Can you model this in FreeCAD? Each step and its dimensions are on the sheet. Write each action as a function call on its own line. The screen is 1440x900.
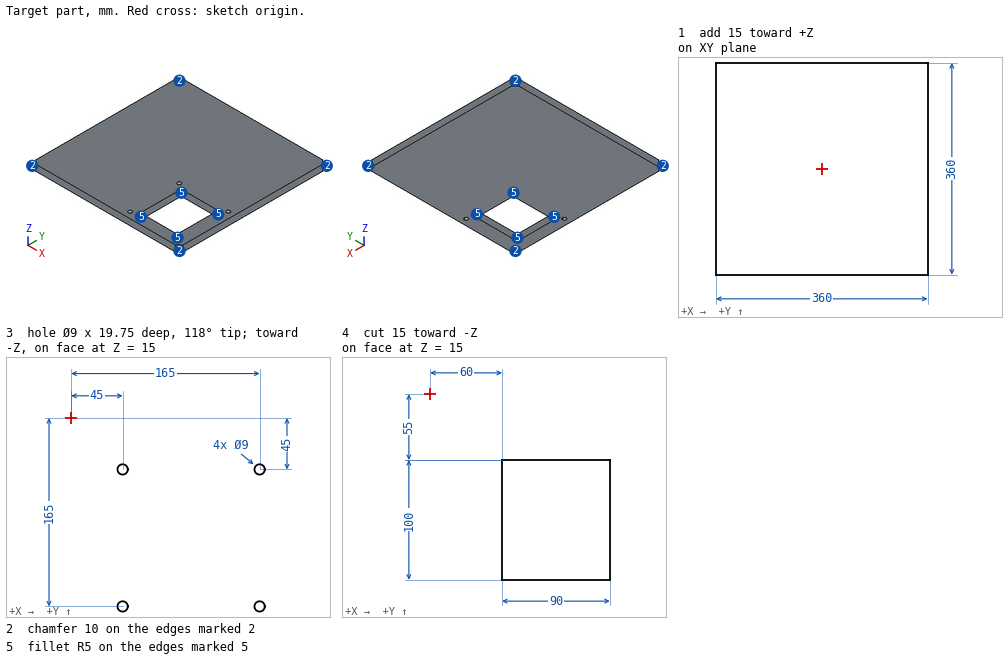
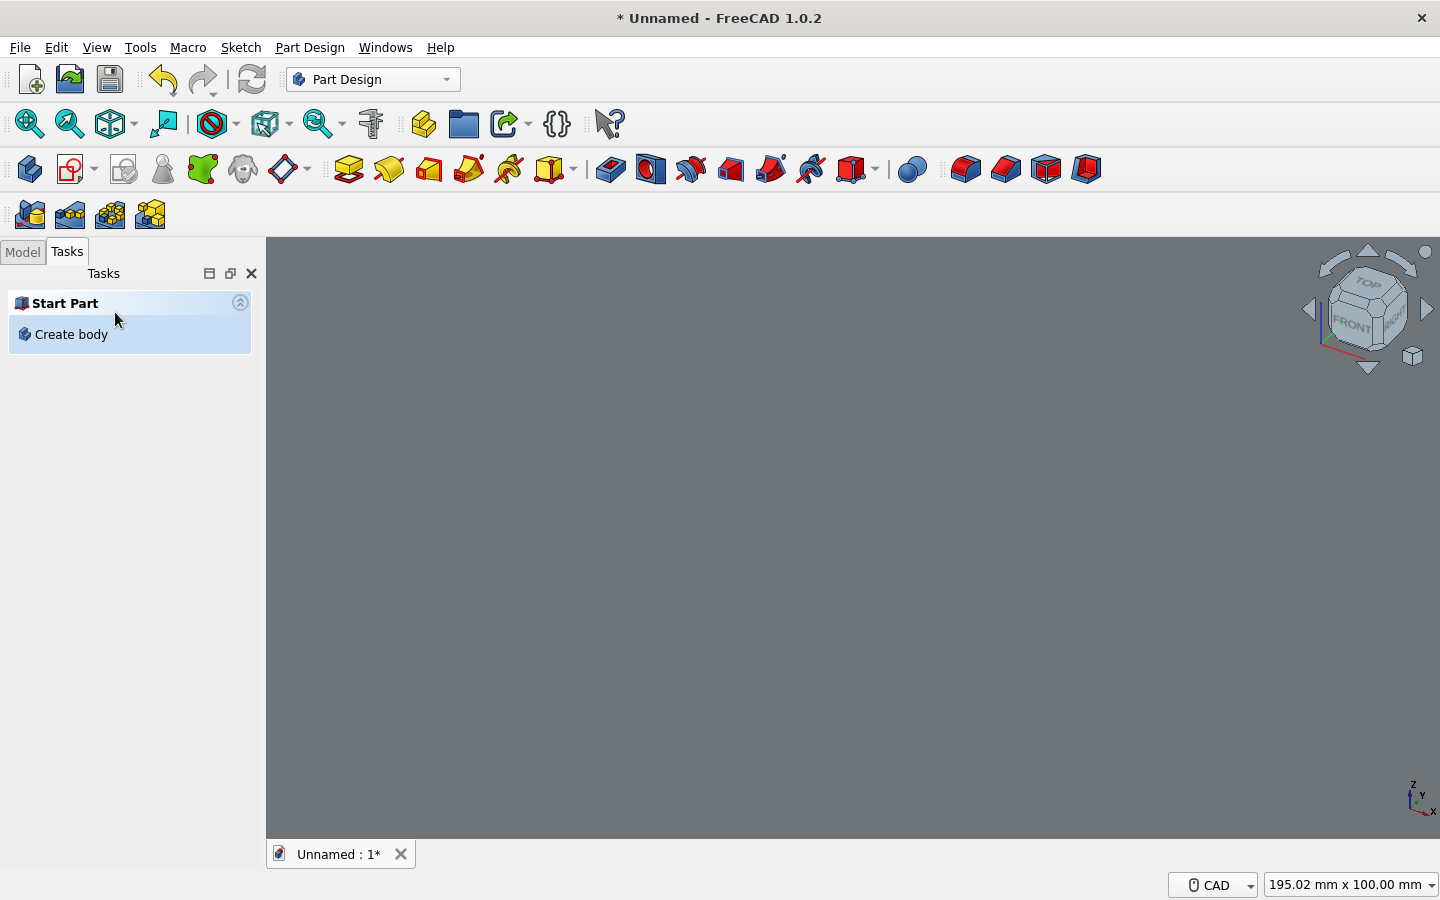
key(v)
key(f)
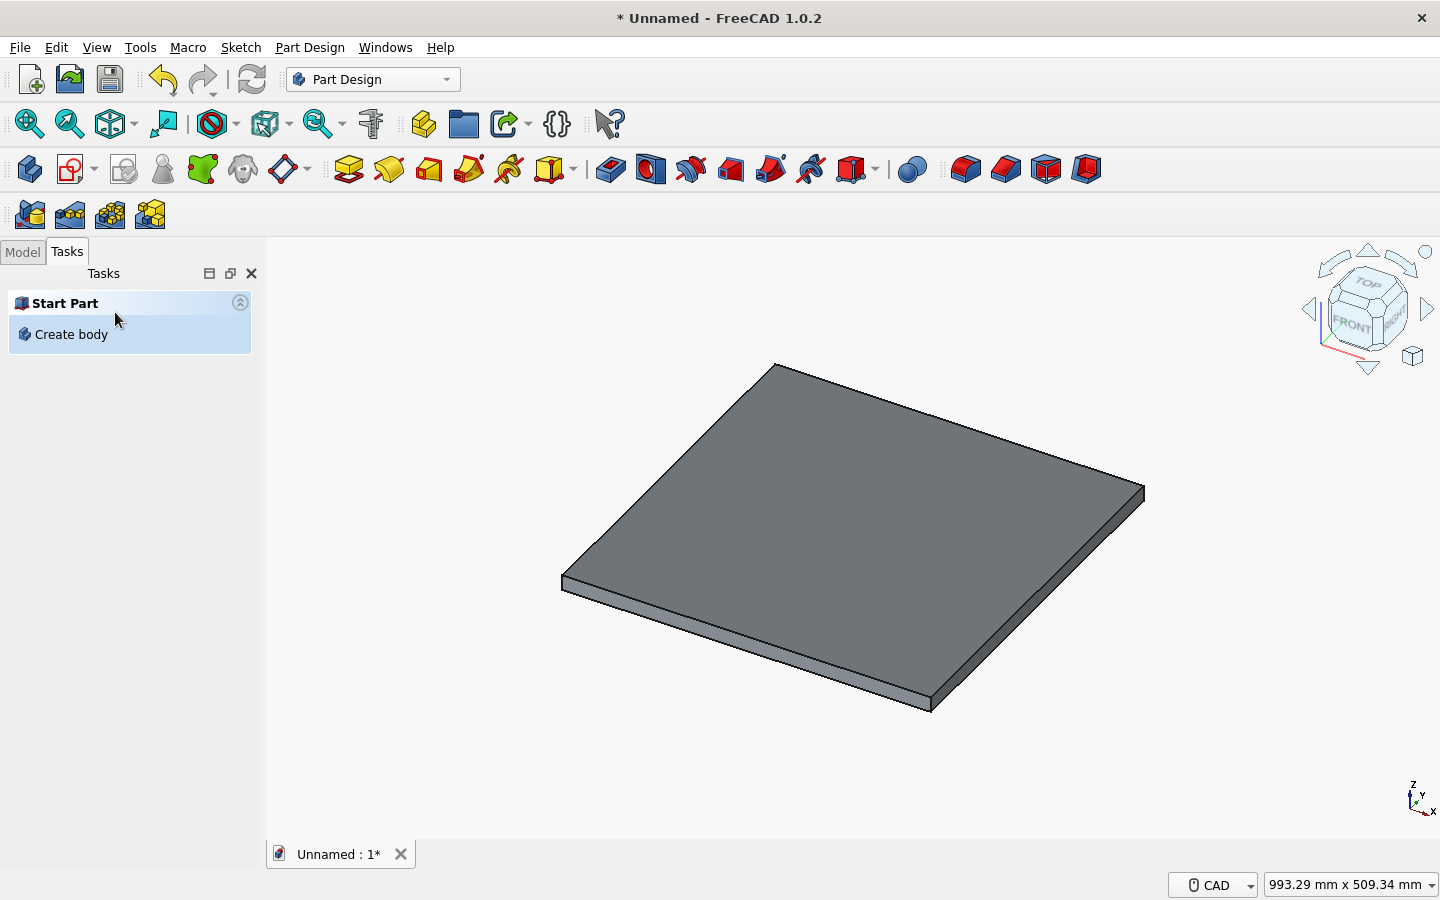
click(931, 704)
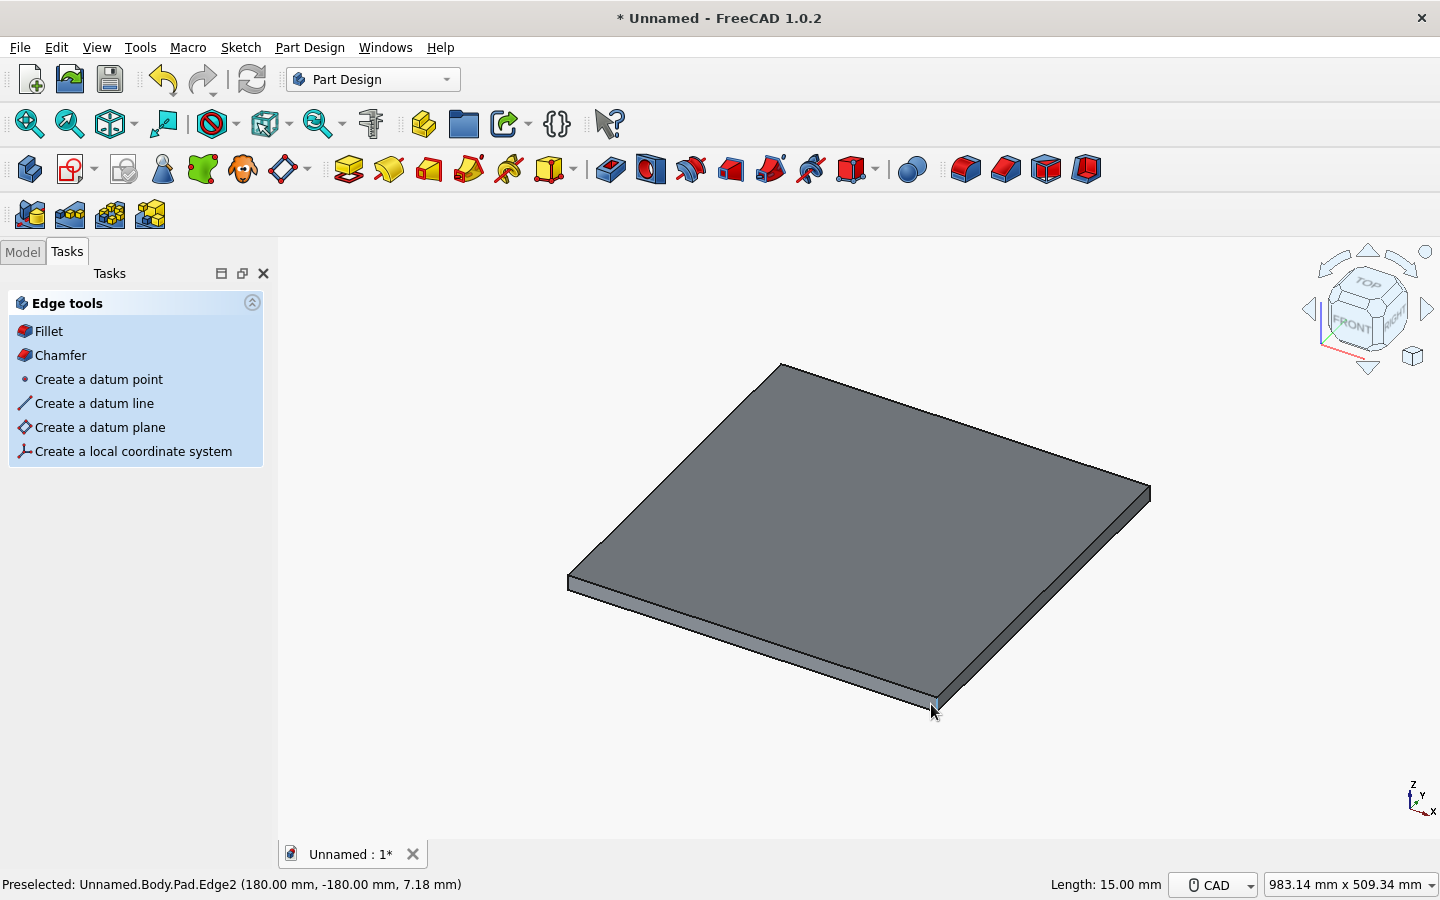
scroll(781, 370, up, 5)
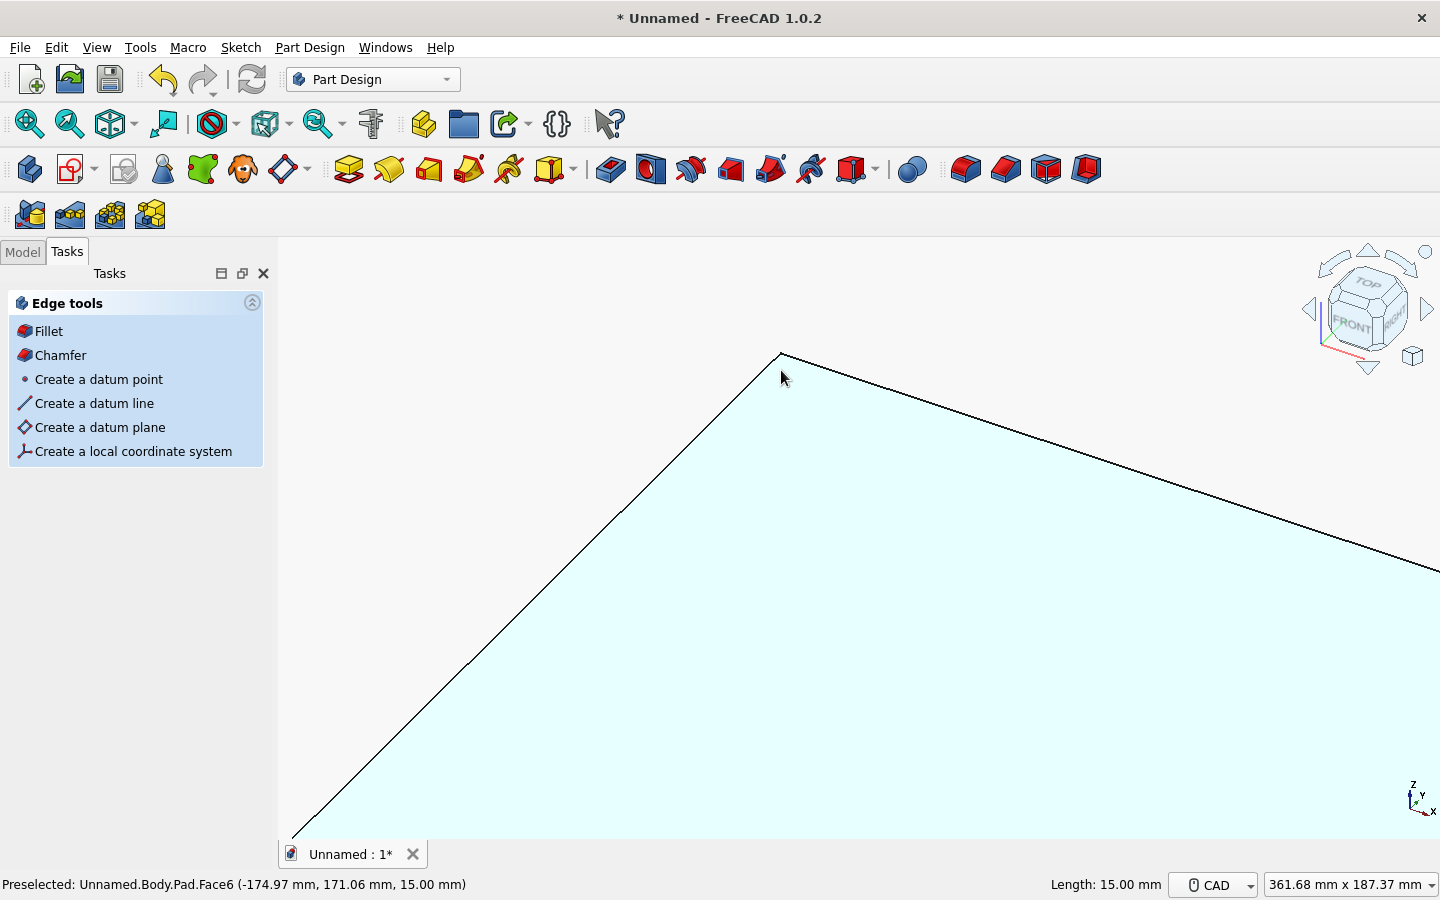
key(v)
key(f)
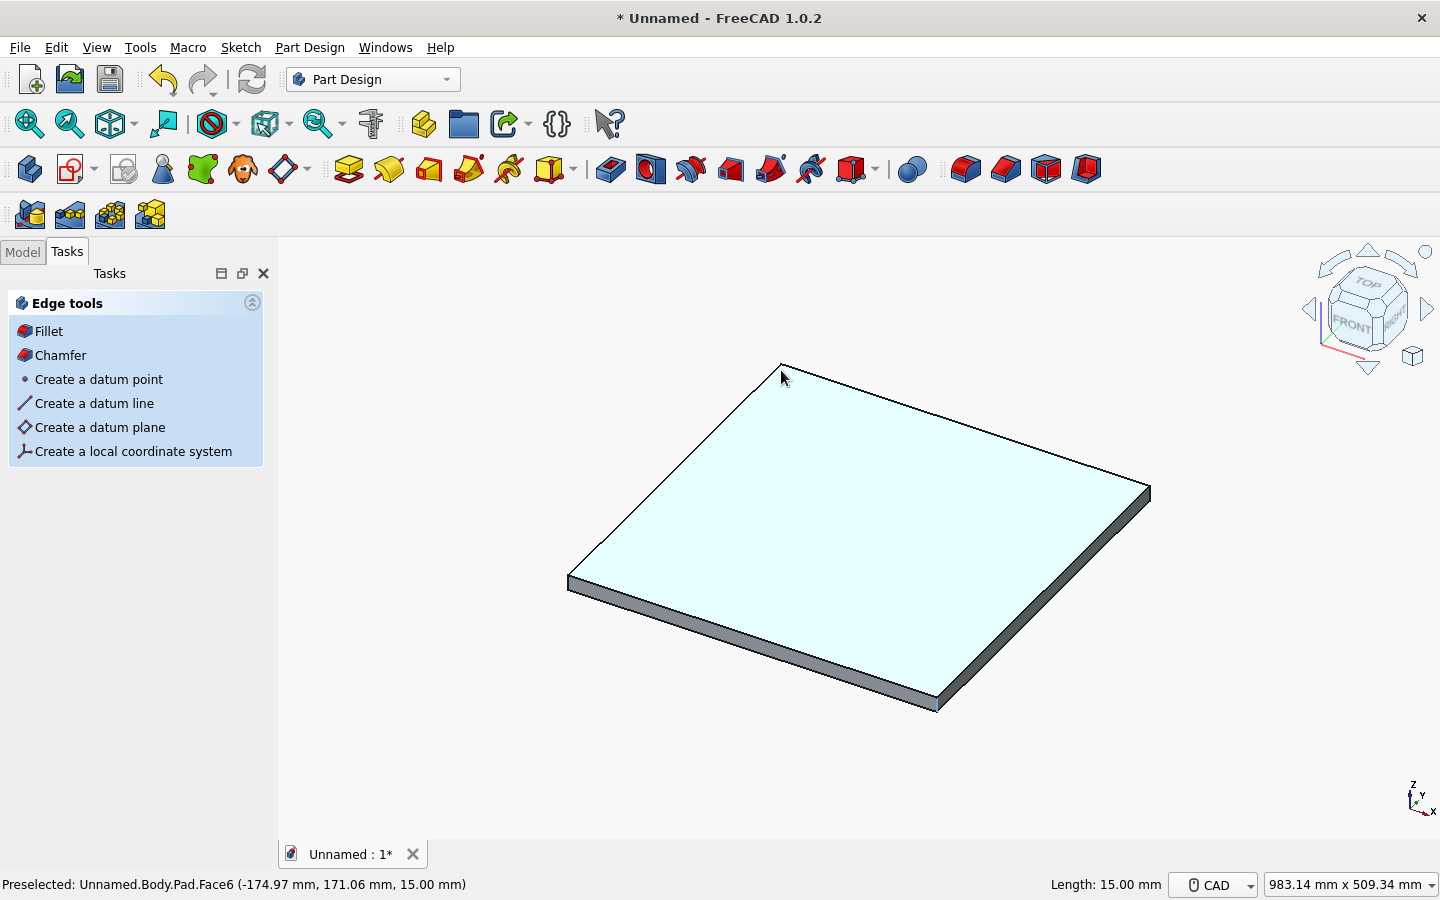
key(0)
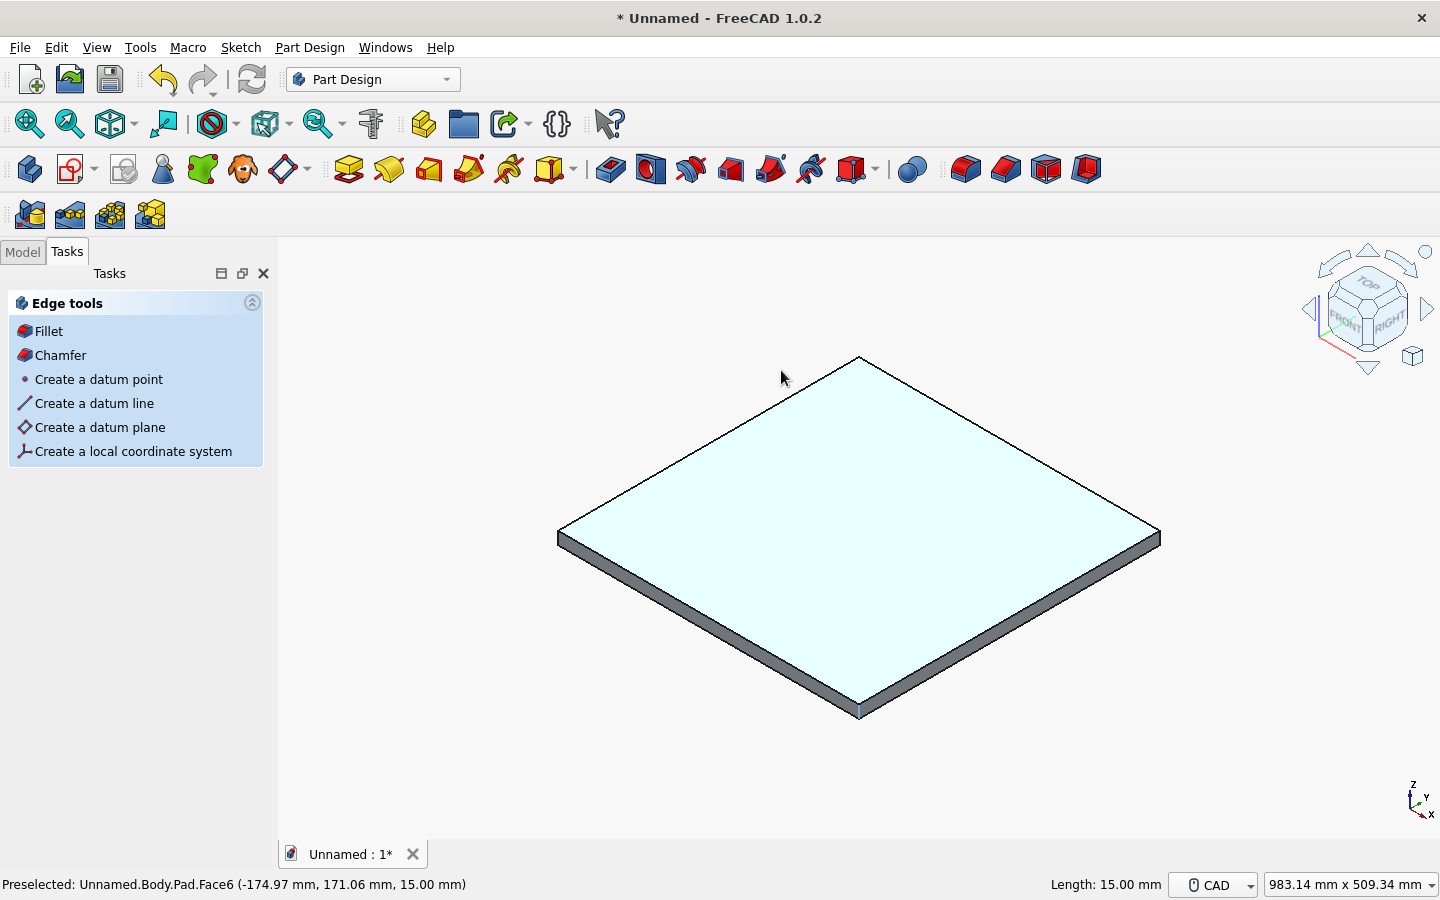
scroll(859, 363, up, 5)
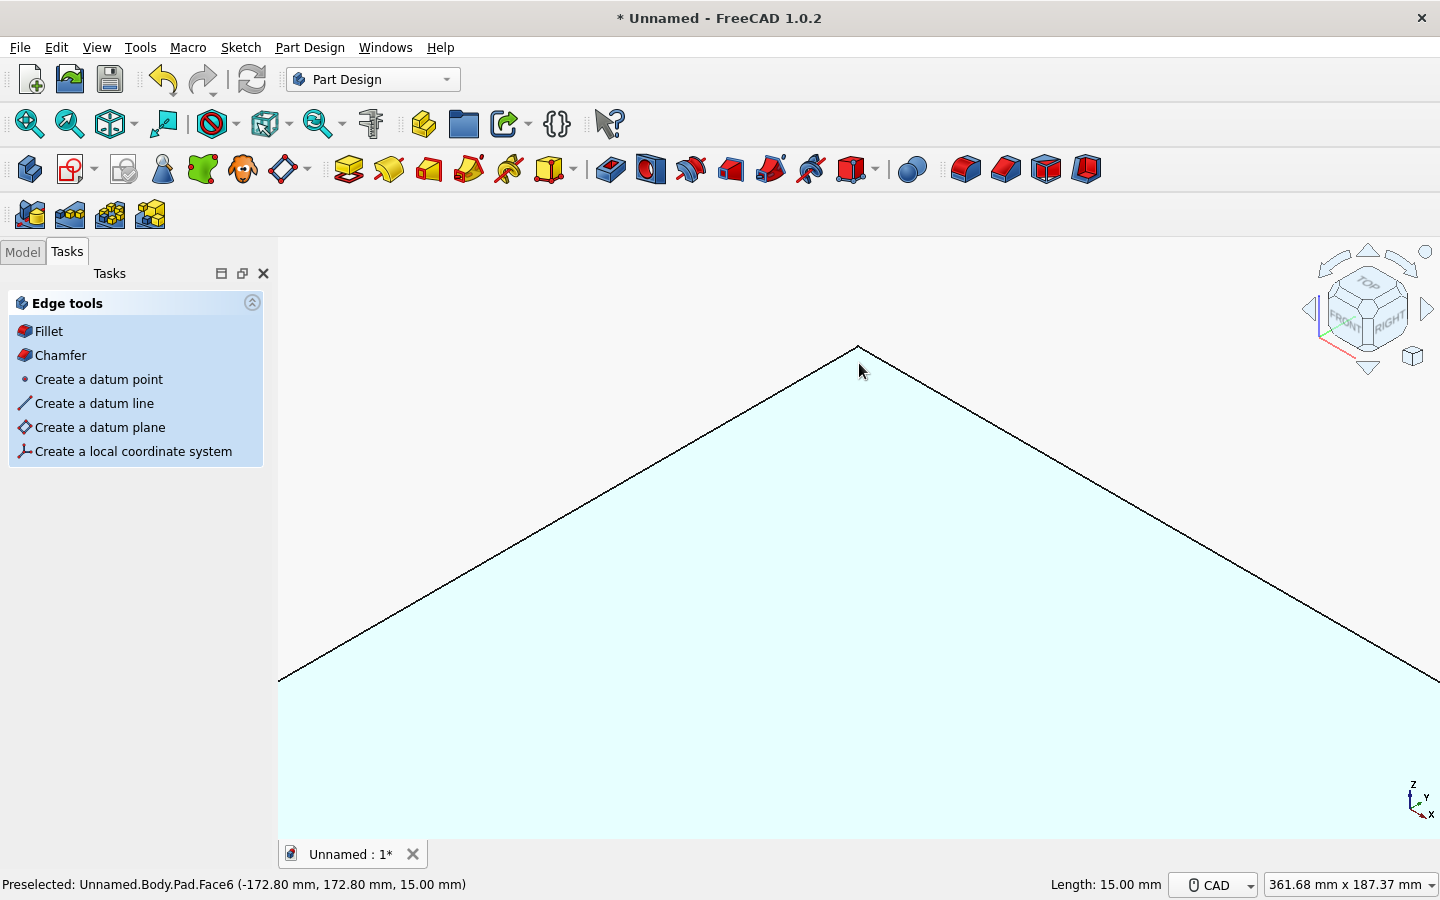
key(v)
key(f)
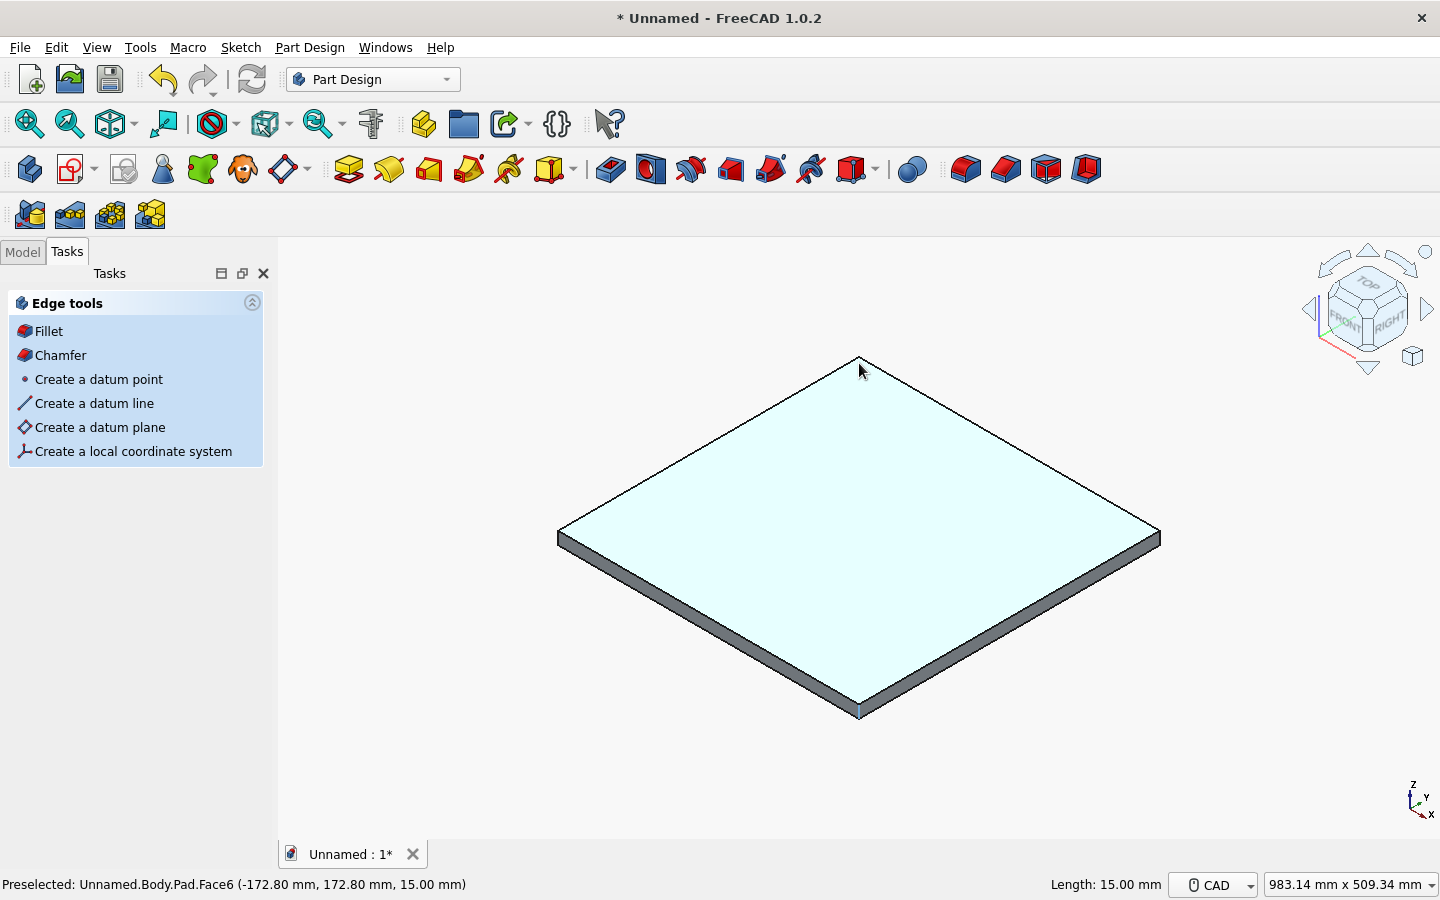
key(2)